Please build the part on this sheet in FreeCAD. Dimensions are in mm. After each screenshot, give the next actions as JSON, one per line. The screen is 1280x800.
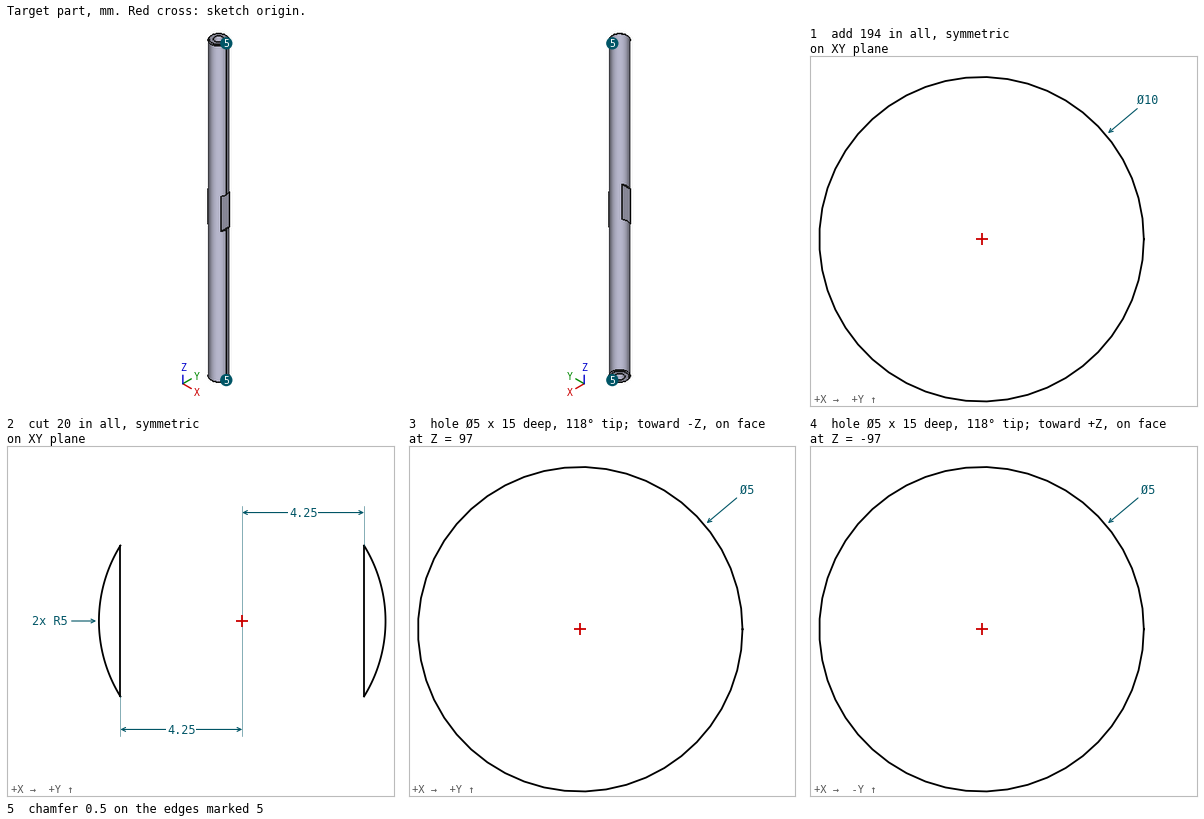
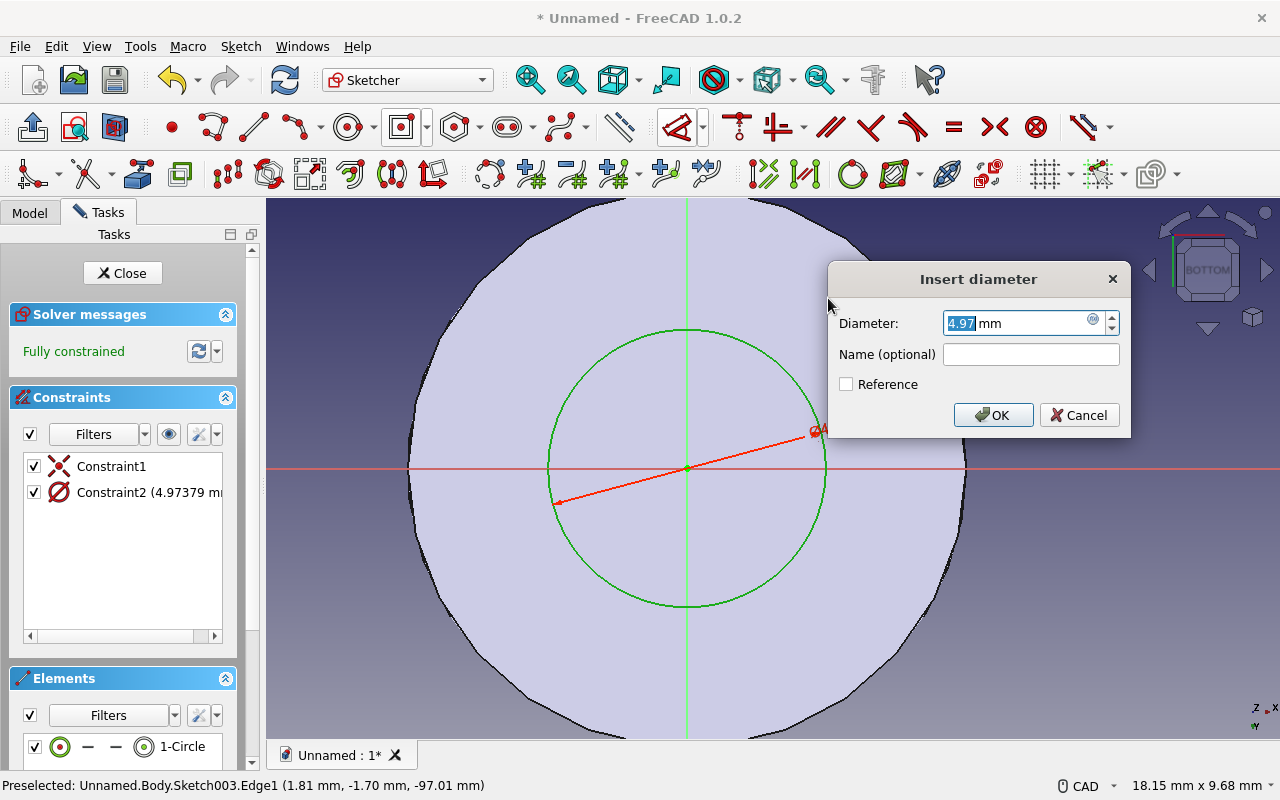
{"action": "type", "text": "5"}
{"action": "key", "text": "Return"}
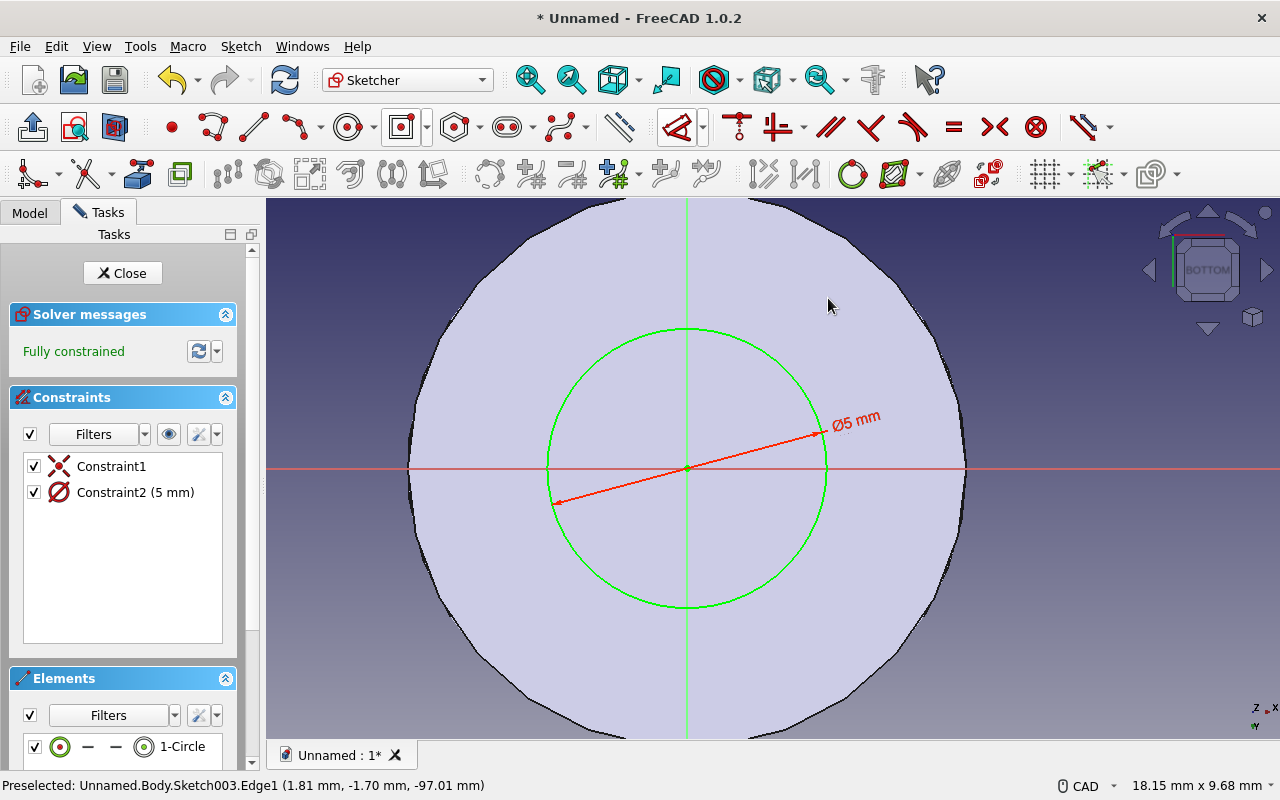
{"action": "left_click", "coordinate": [123, 273]}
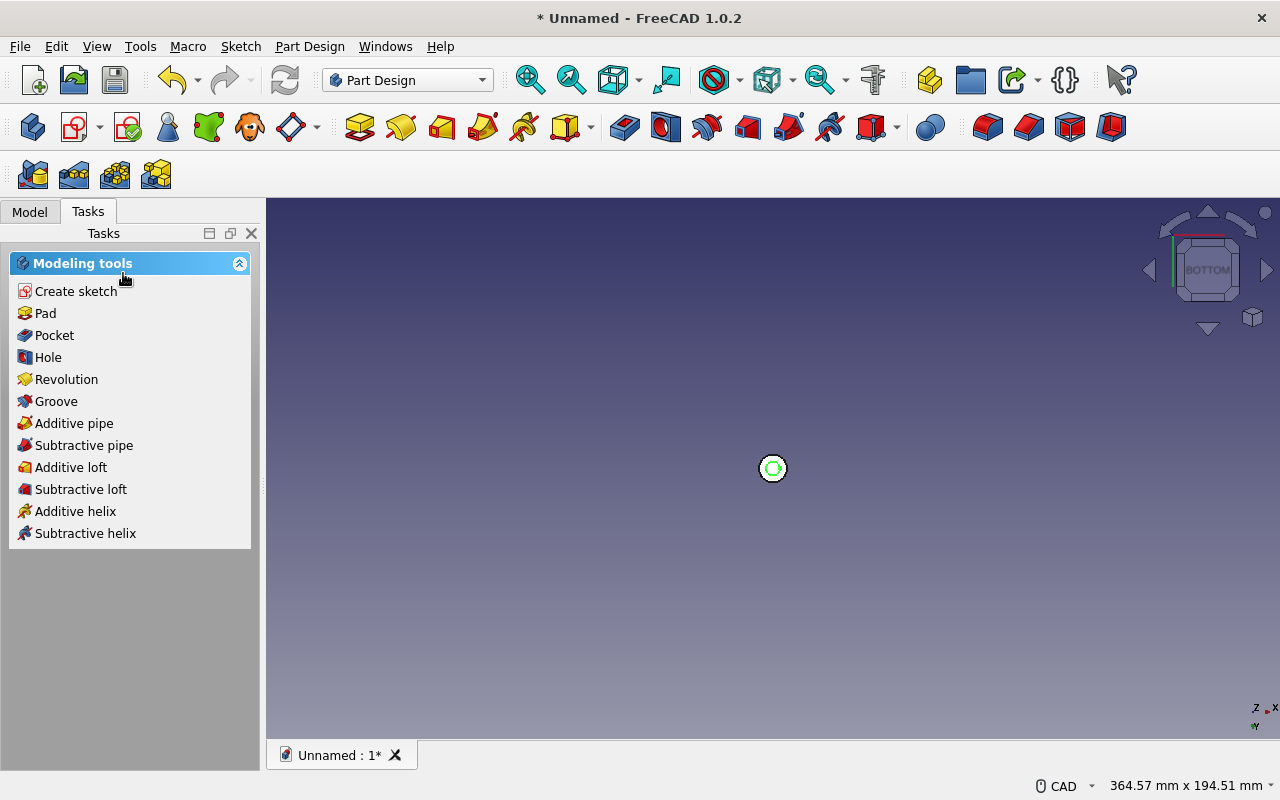
{"action": "left_click", "coordinate": [666, 128]}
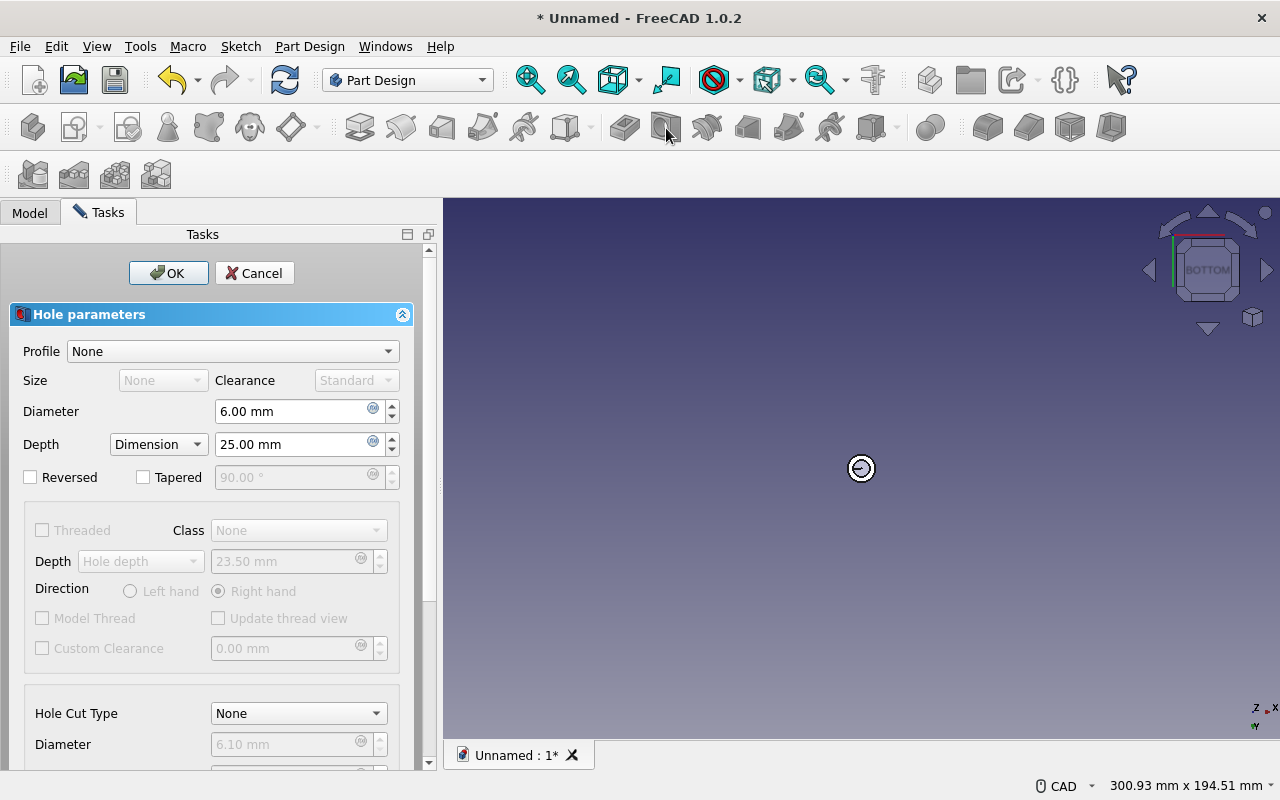
{"action": "triple_click", "coordinate": [300, 412]}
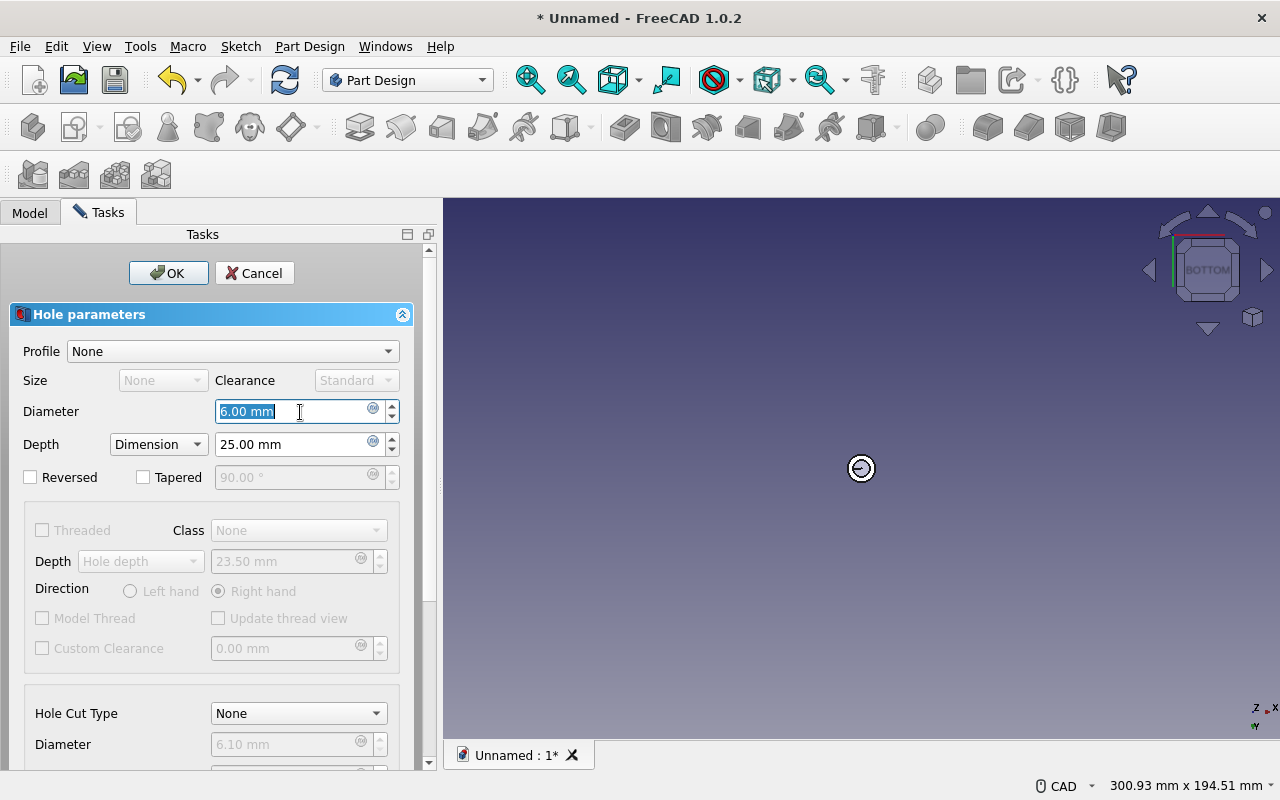
{"action": "type", "text": "5"}
{"action": "key", "text": "Tab"}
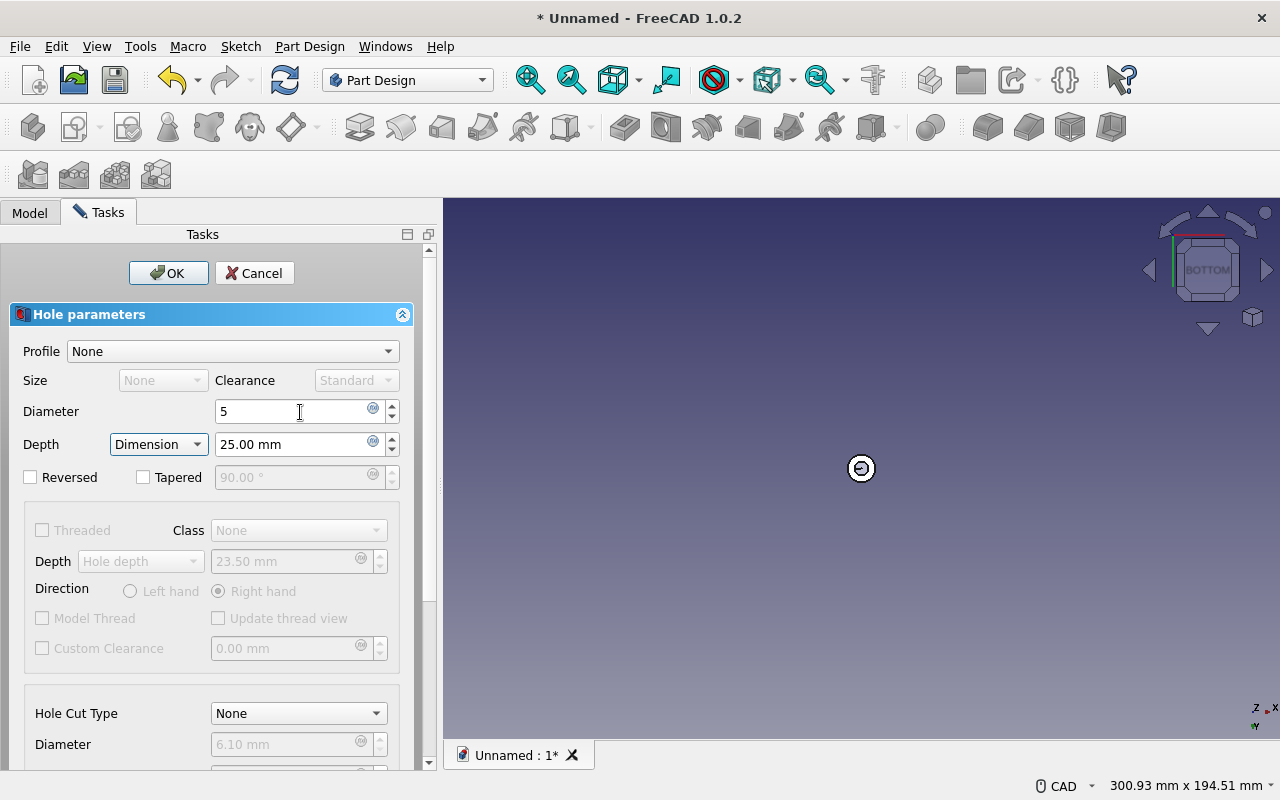
{"action": "triple_click", "coordinate": [300, 444]}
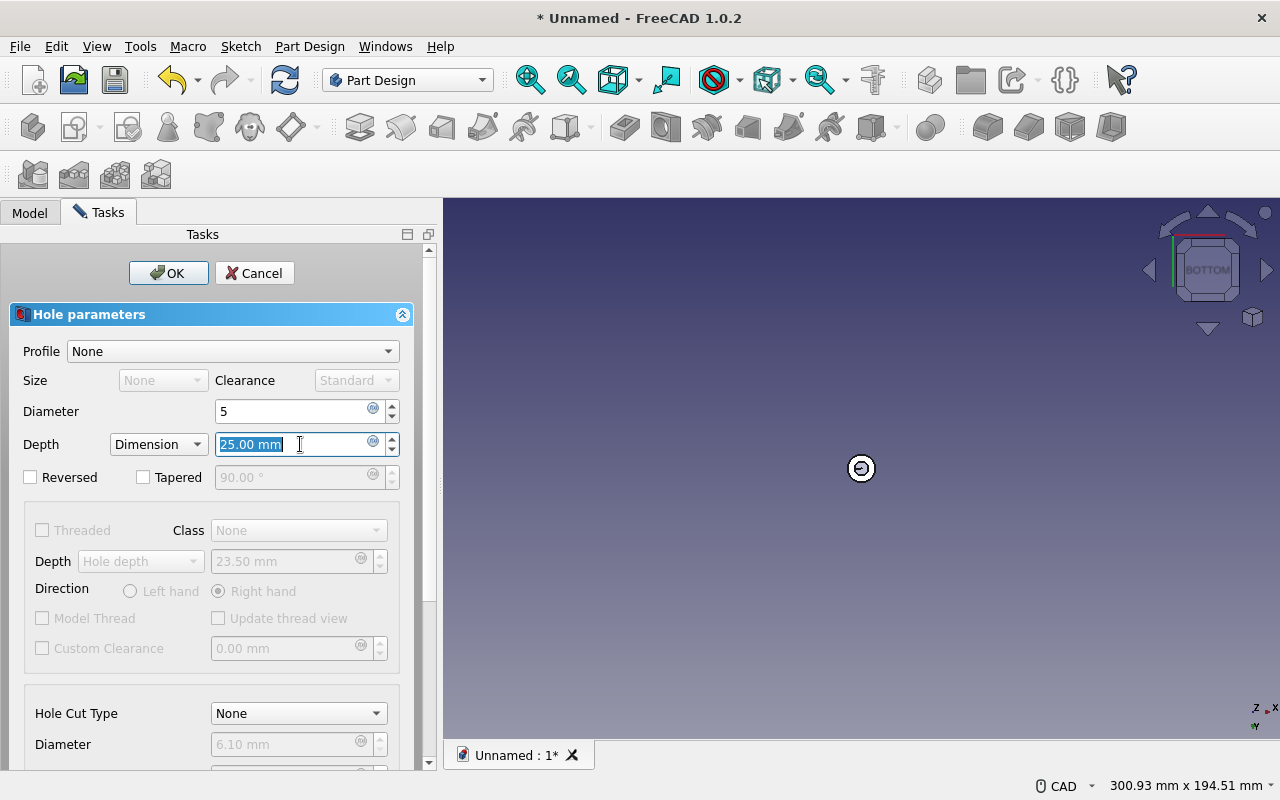
{"action": "type", "text": "15"}
{"action": "key", "text": "Tab"}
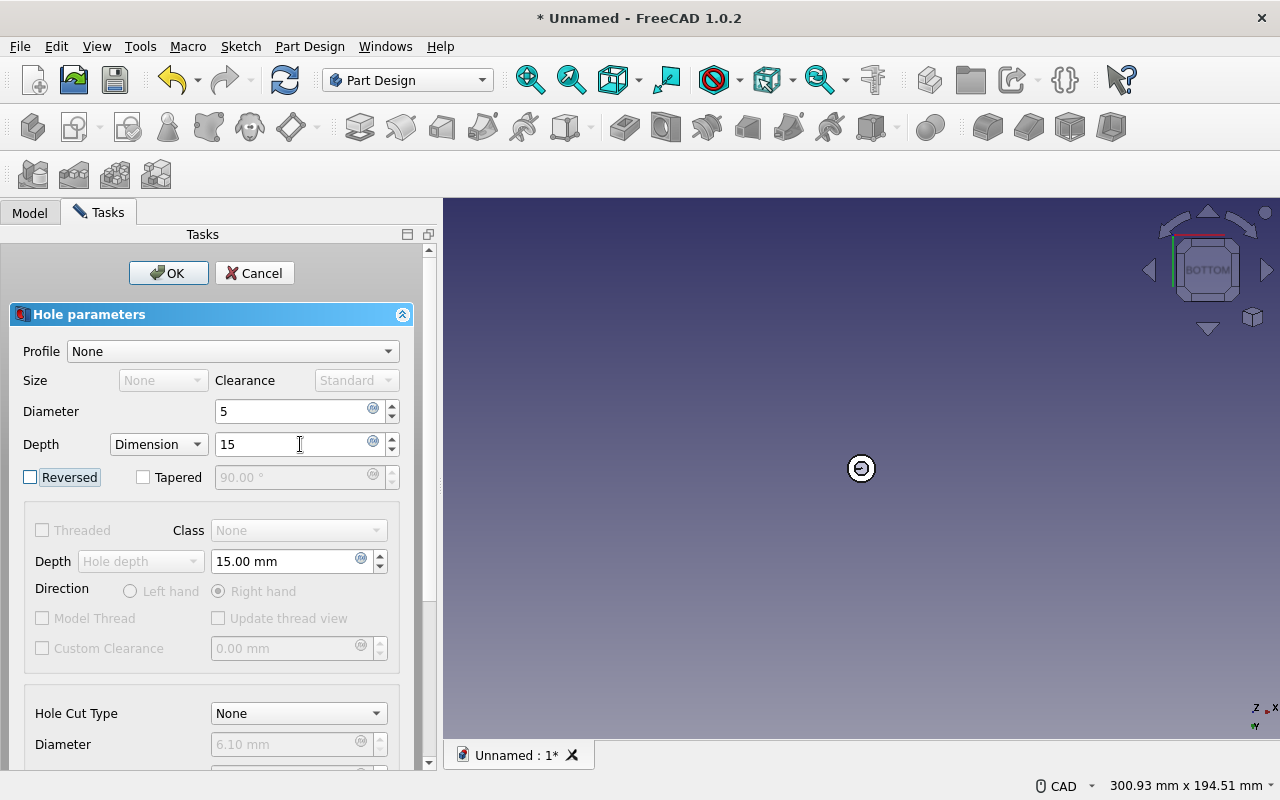
{"action": "left_click", "coordinate": [169, 273]}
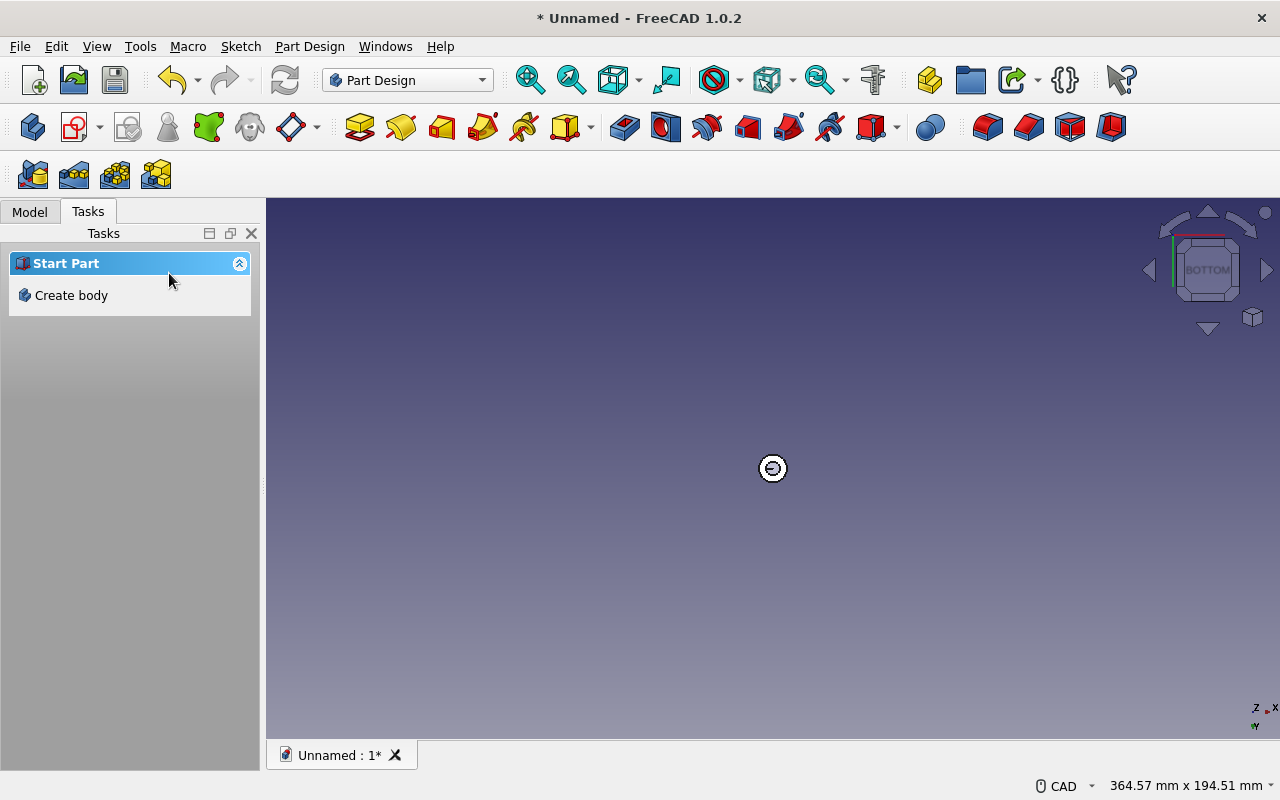
{"action": "left_click", "coordinate": [531, 80]}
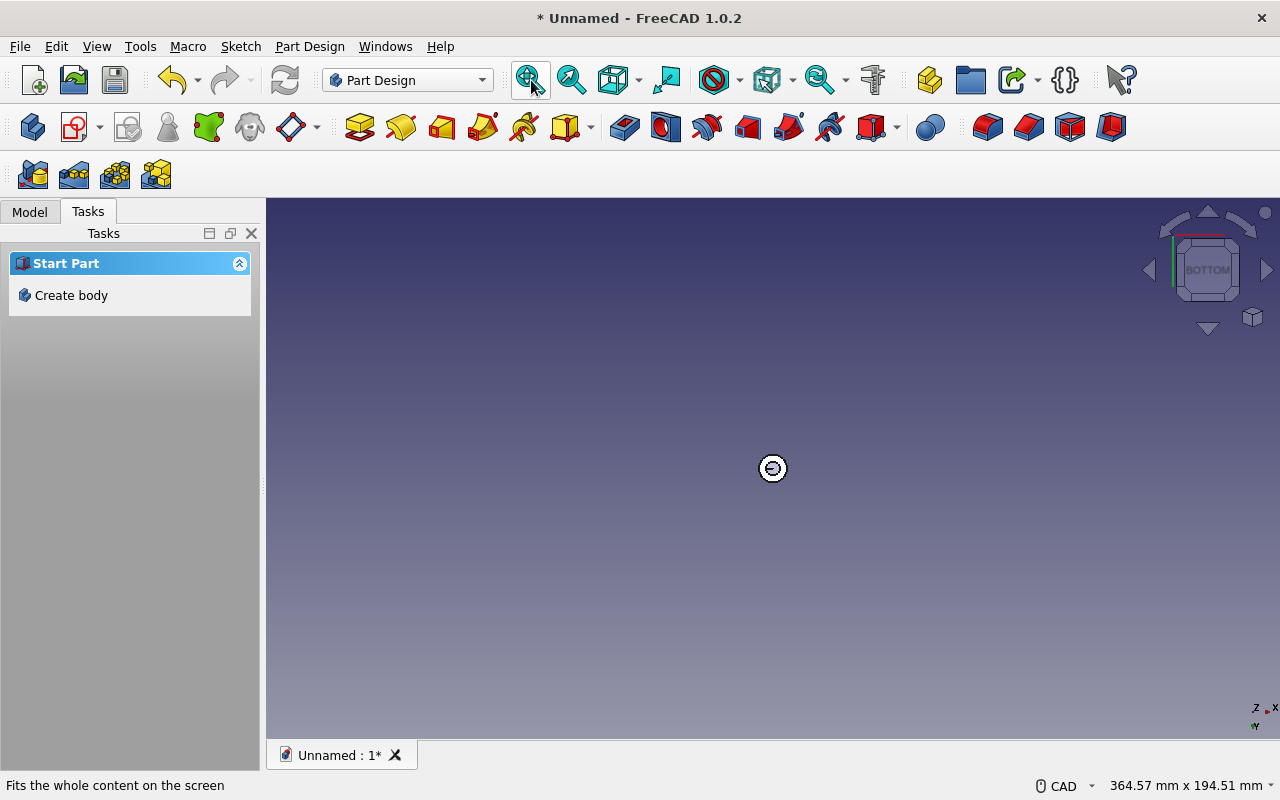
{"action": "left_click", "coordinate": [759, 467]}